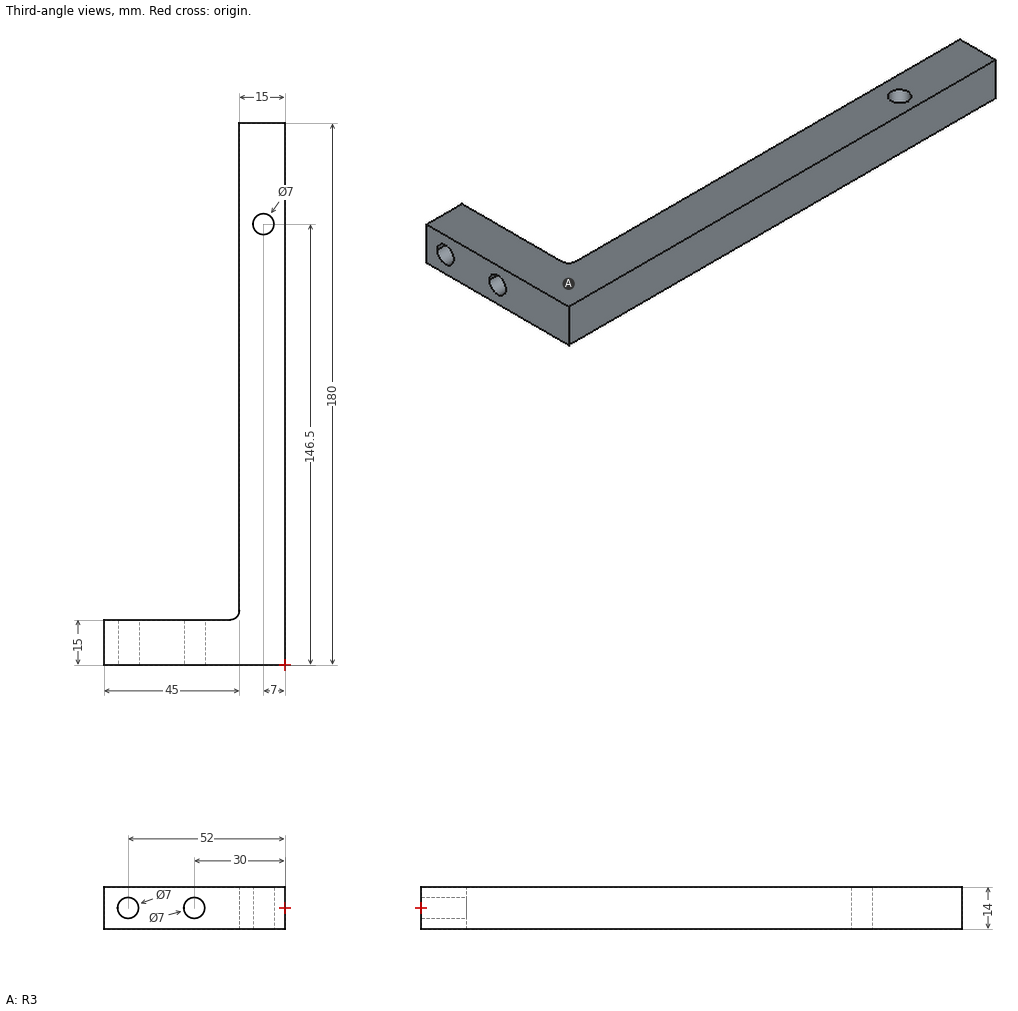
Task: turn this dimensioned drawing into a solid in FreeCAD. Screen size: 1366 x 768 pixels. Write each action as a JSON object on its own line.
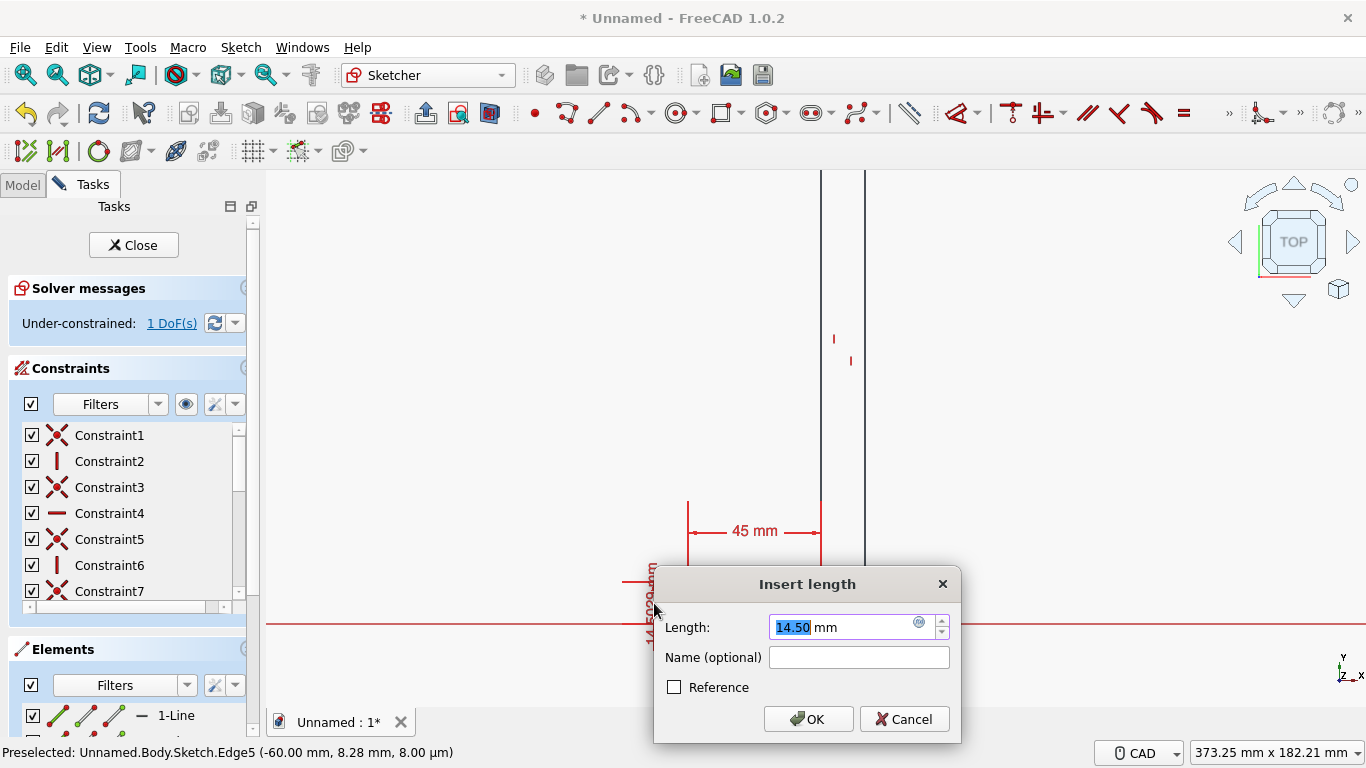
{"action": "type", "text": "15"}
{"action": "key", "text": "Return"}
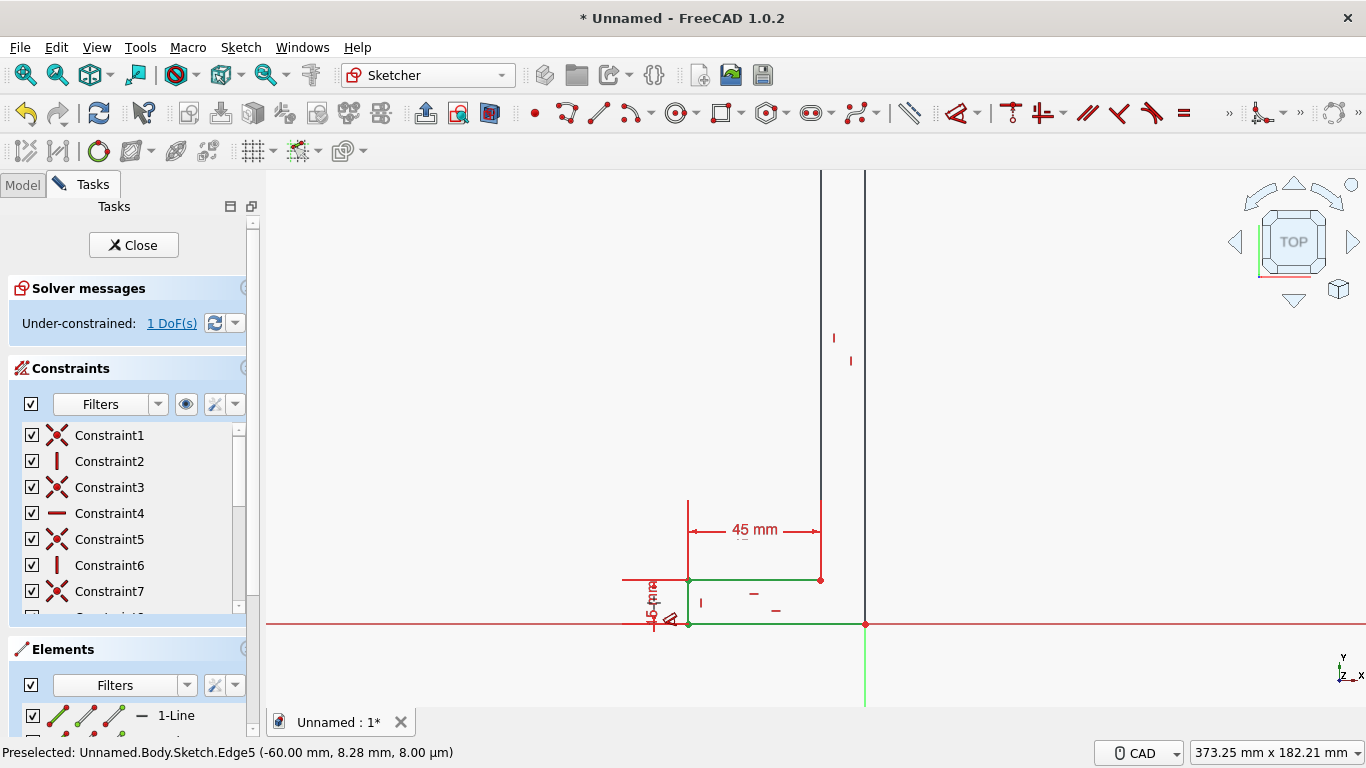
{"action": "left_click", "coordinate": [865, 466]}
{"action": "left_click", "coordinate": [899, 411]}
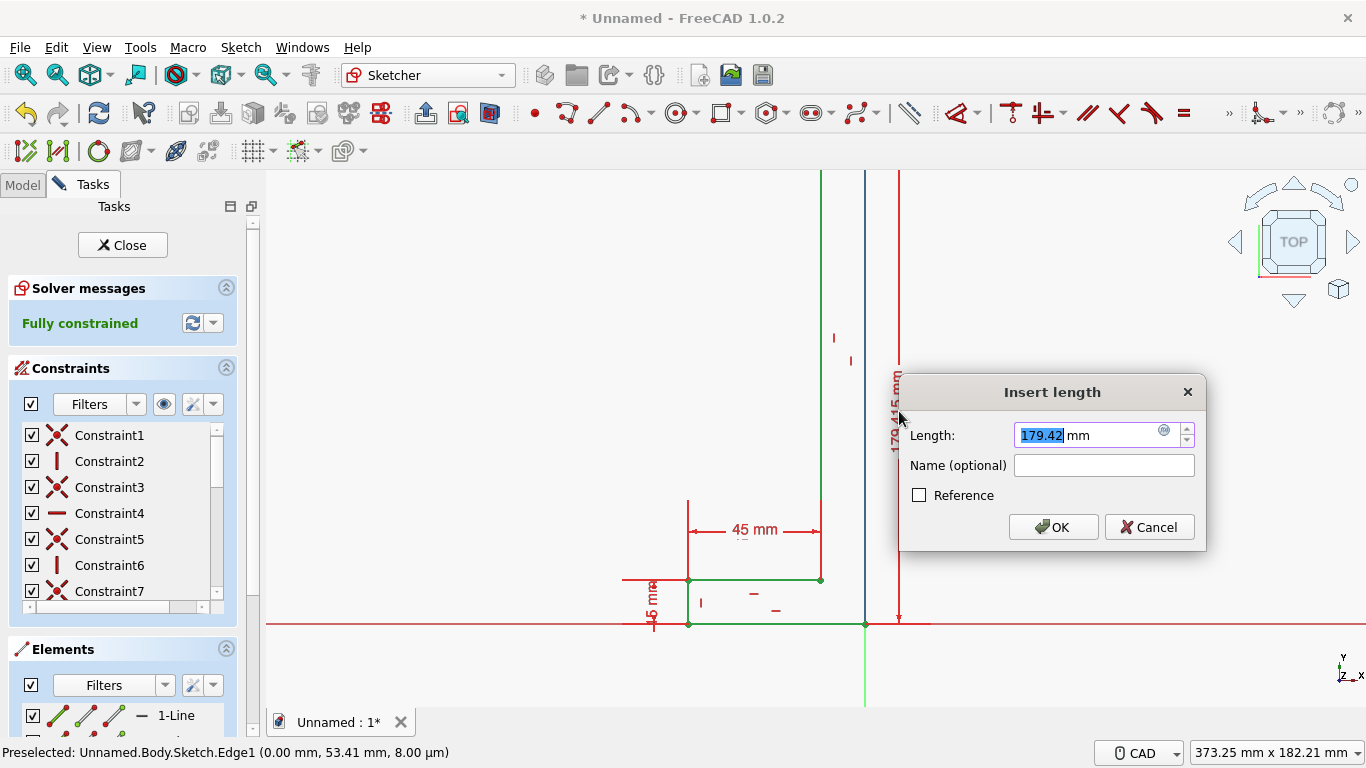
{"action": "type", "text": "180"}
{"action": "key", "text": "Return"}
{"action": "key", "text": "Escape"}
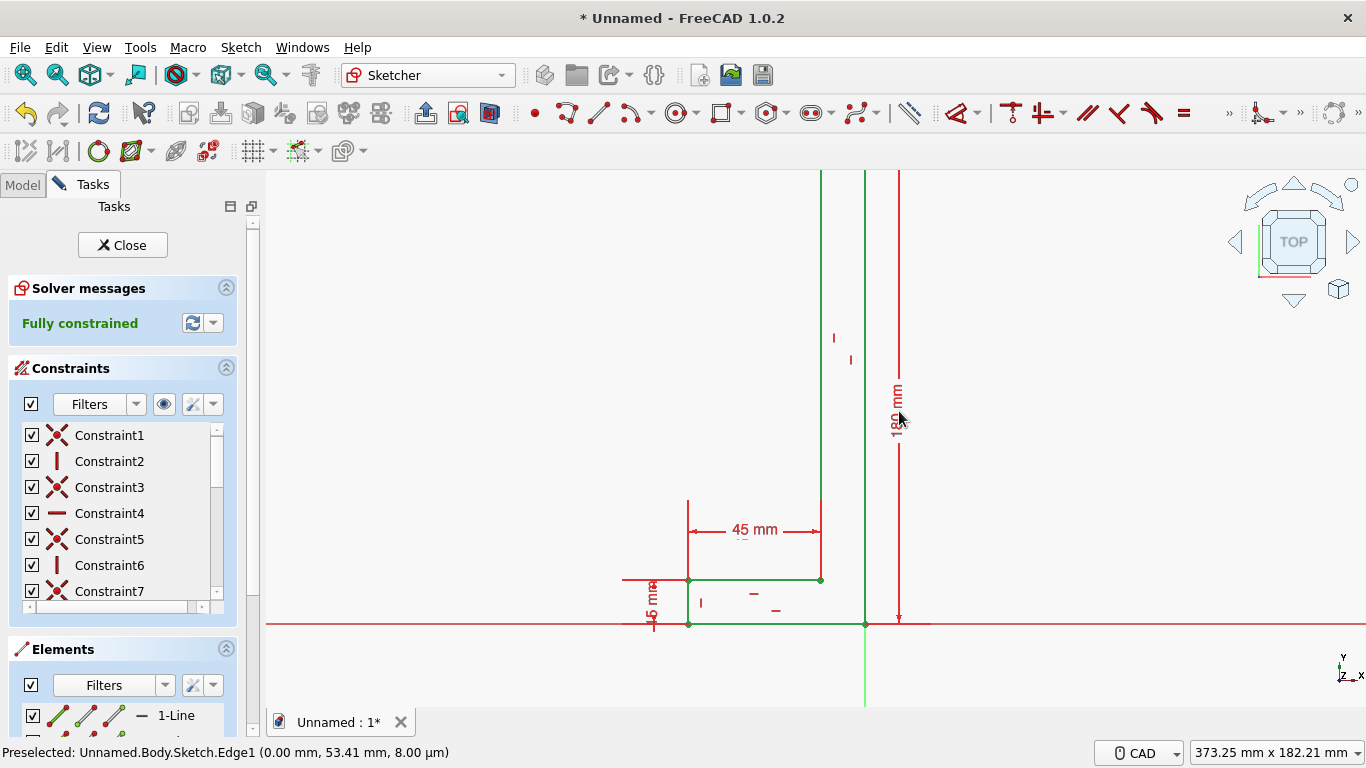
{"action": "left_click", "coordinate": [123, 245]}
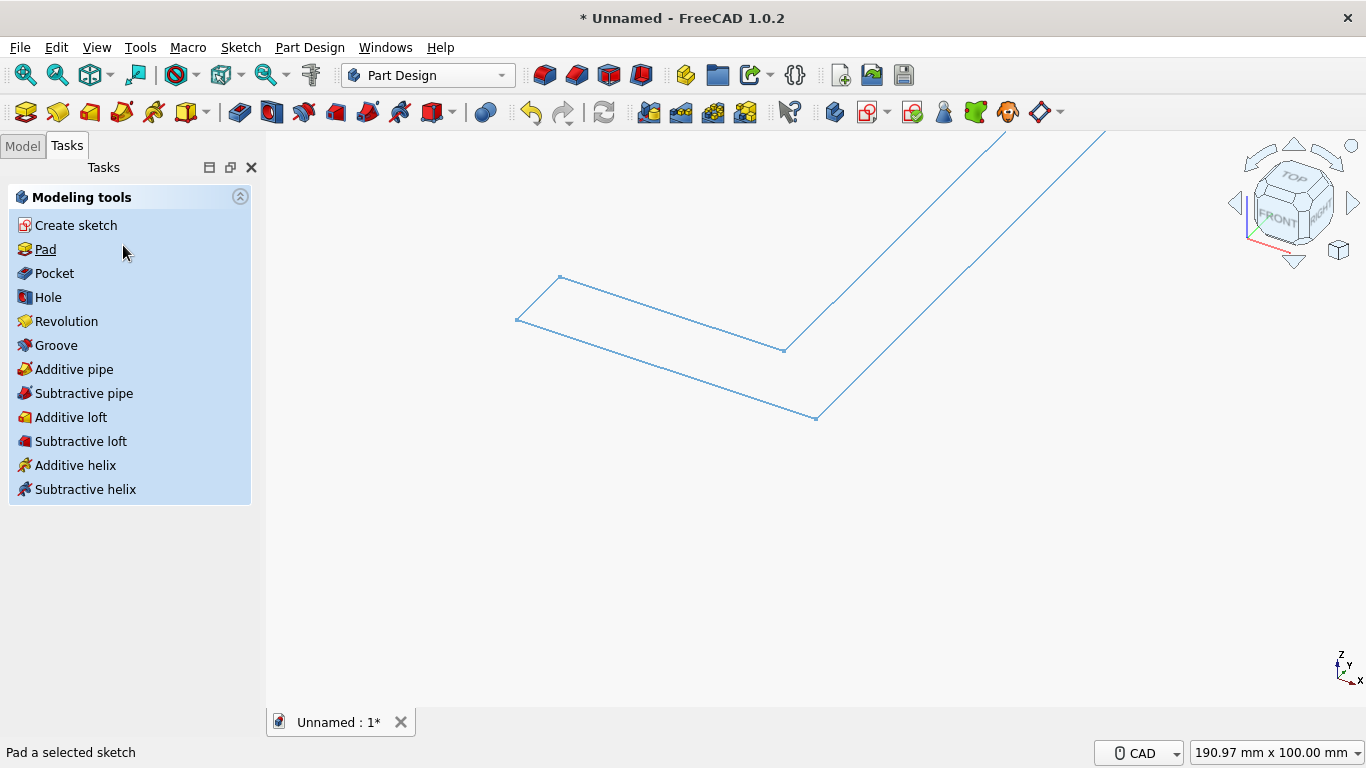
{"action": "left_click", "coordinate": [26, 112]}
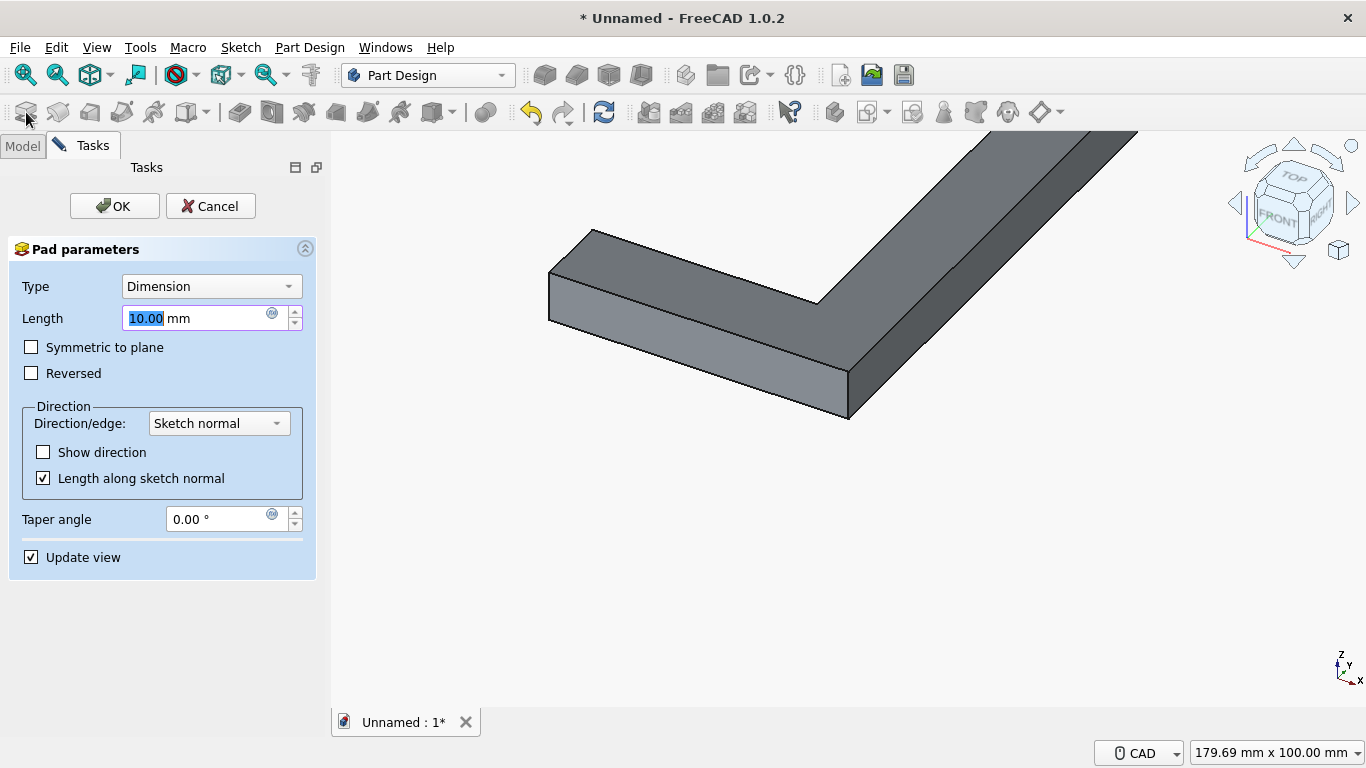
{"action": "type", "text": "14"}
{"action": "key", "text": "Tab"}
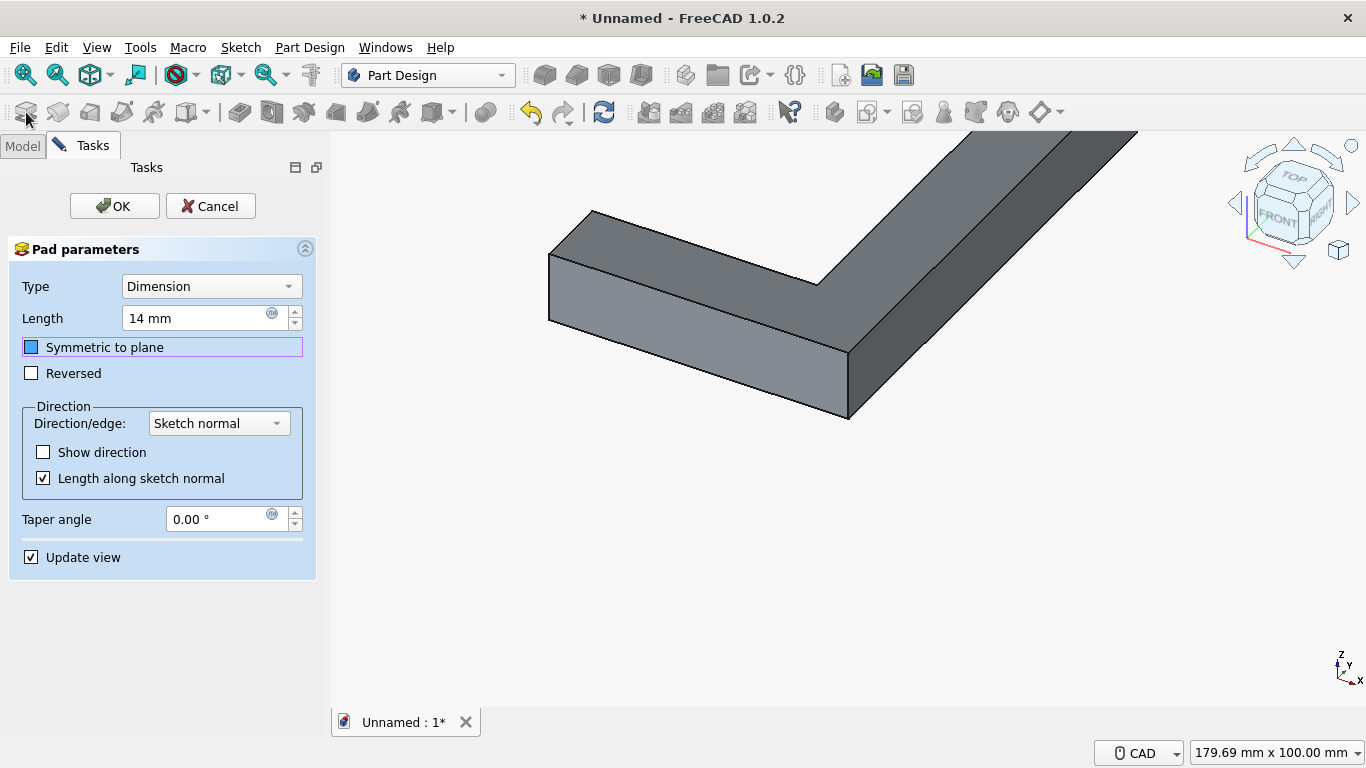
{"action": "left_click", "coordinate": [30, 347]}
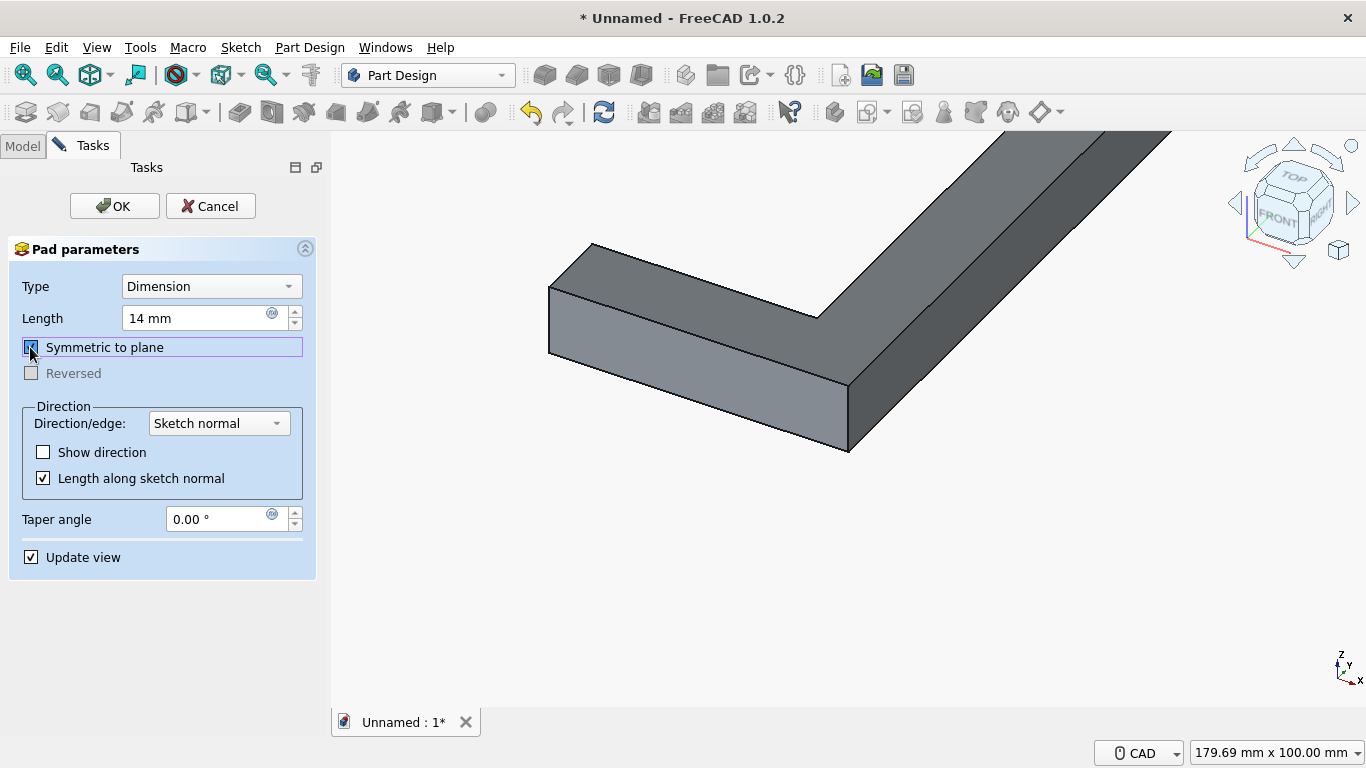
{"action": "left_click", "coordinate": [115, 206]}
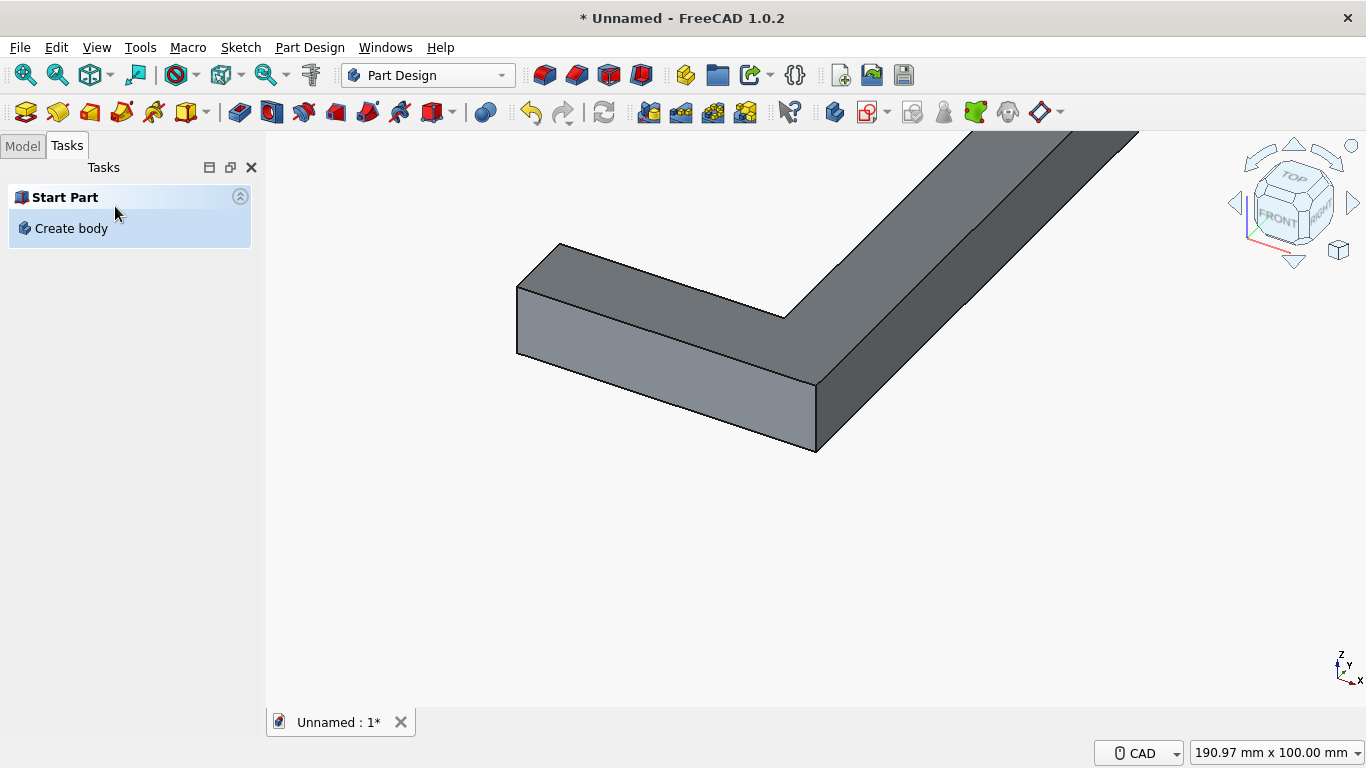
{"action": "left_click", "coordinate": [26, 76]}